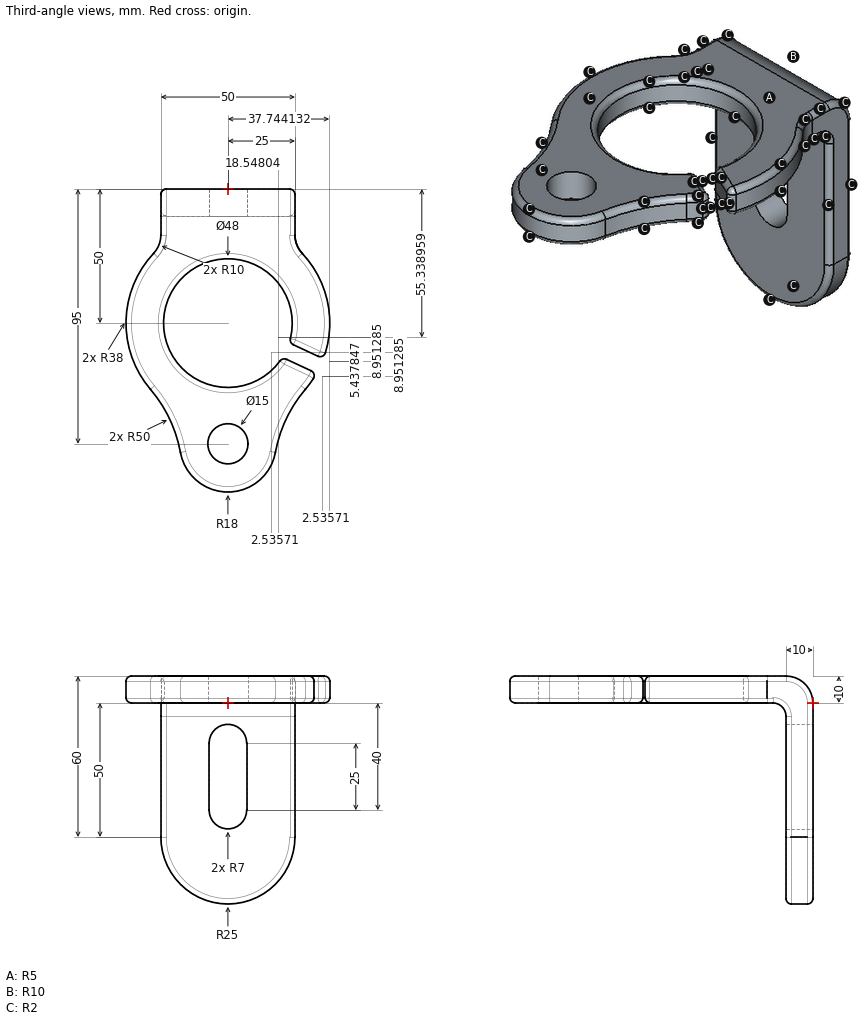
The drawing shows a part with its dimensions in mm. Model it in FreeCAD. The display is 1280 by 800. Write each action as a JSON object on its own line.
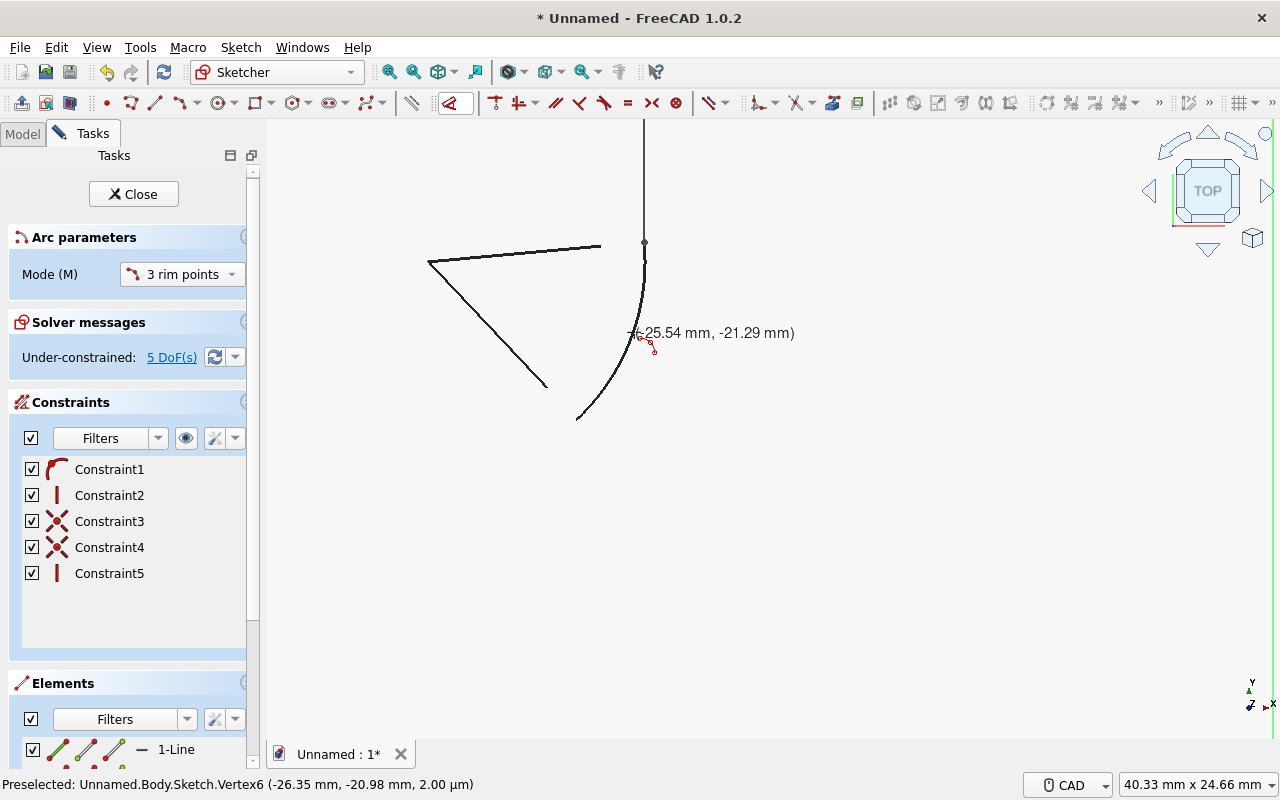
{"action": "left_click", "coordinate": [627, 327]}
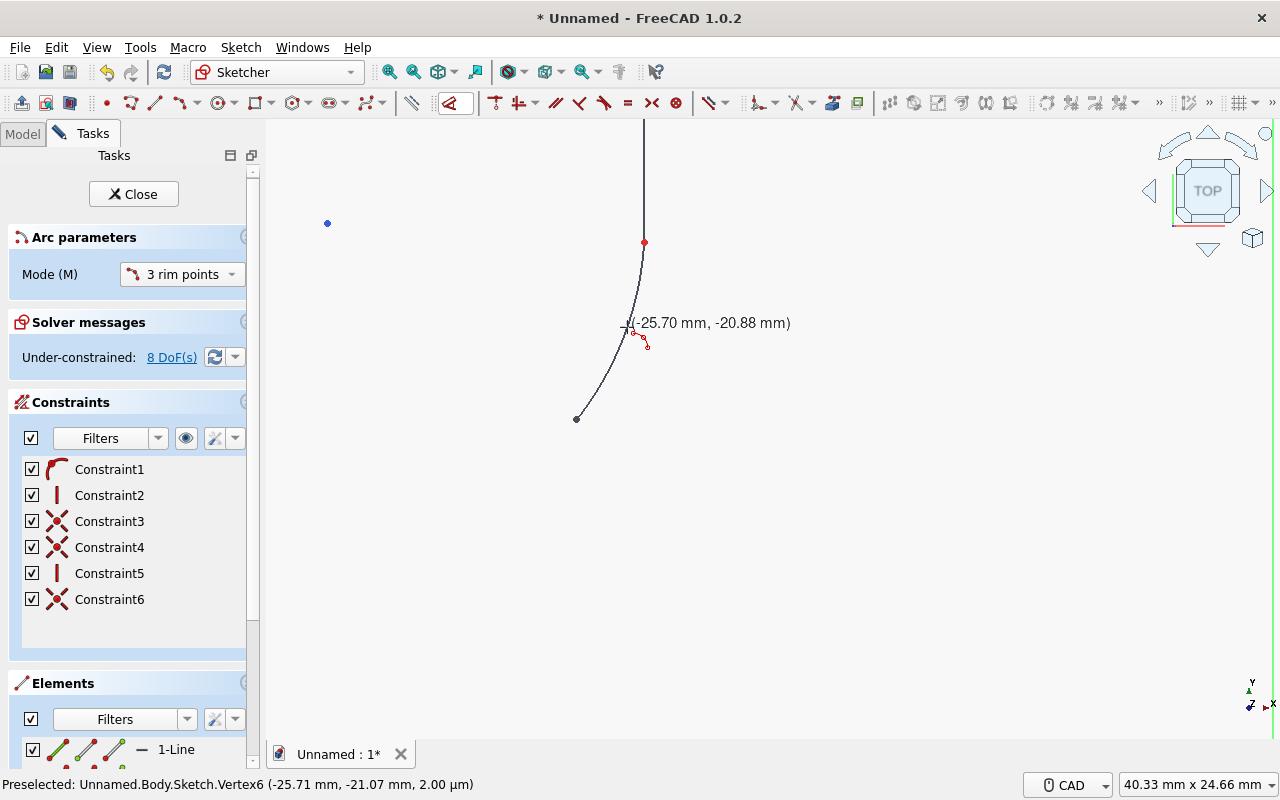
{"action": "scroll", "coordinate": [615, 305], "scroll_direction": "down", "scroll_amount": 10}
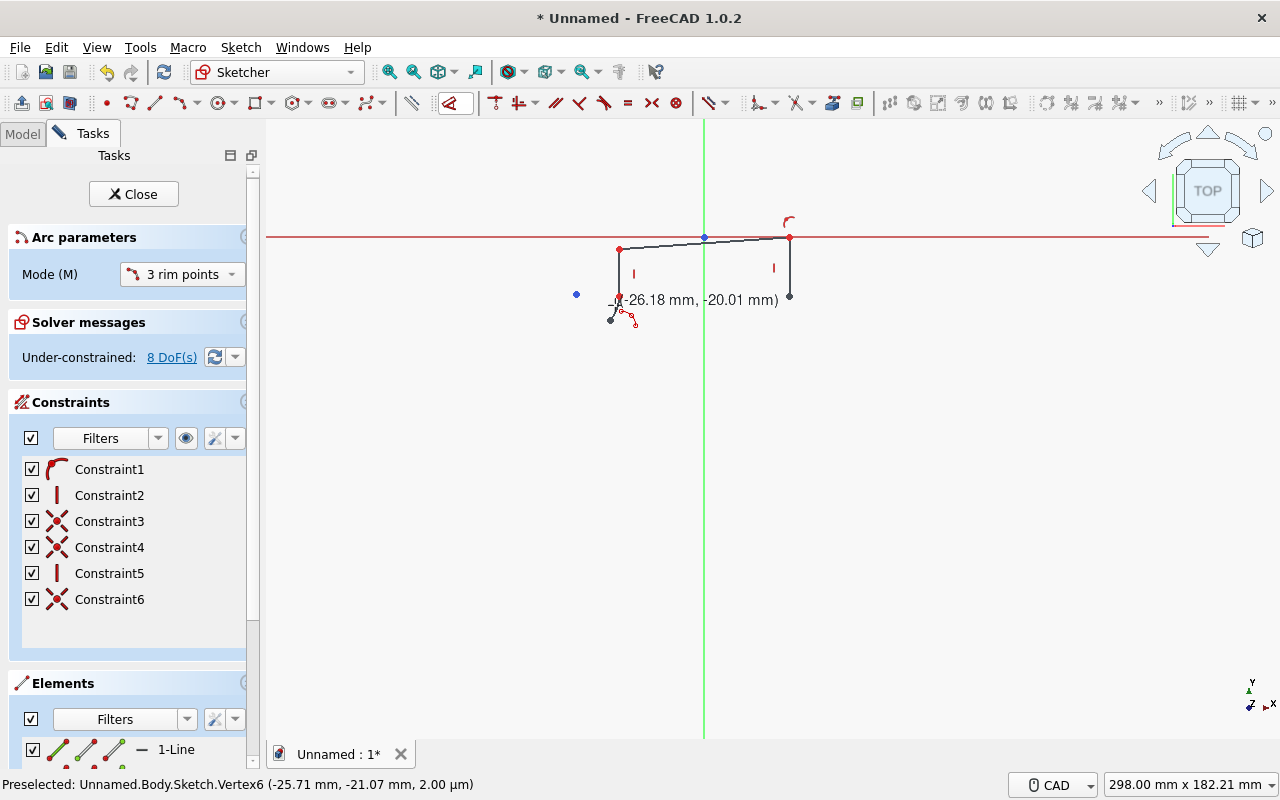
{"action": "left_click", "coordinate": [610, 321]}
{"action": "left_click", "coordinate": [606, 491]}
{"action": "left_click", "coordinate": [575, 404]}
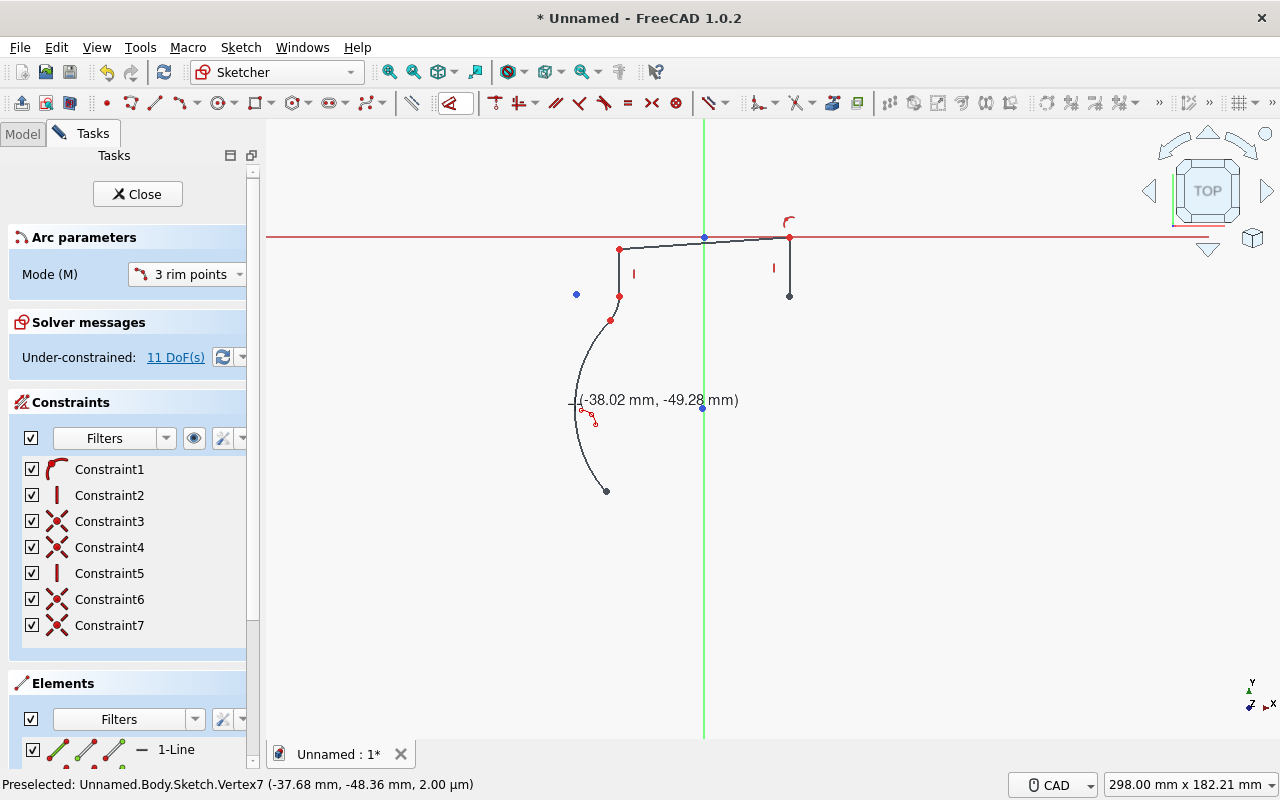
{"action": "left_click", "coordinate": [606, 492]}
{"action": "left_click", "coordinate": [644, 572]}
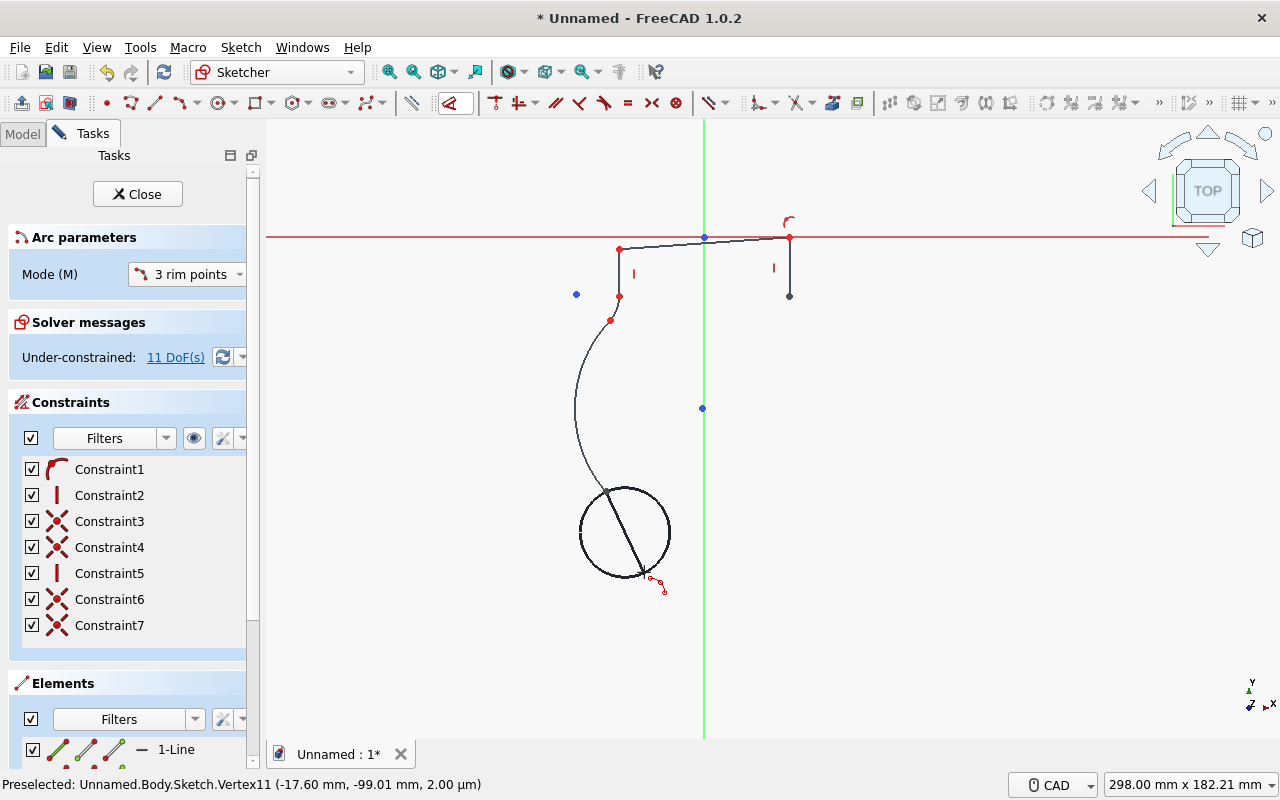
{"action": "scroll", "coordinate": [630, 529], "scroll_direction": "up", "scroll_amount": 5}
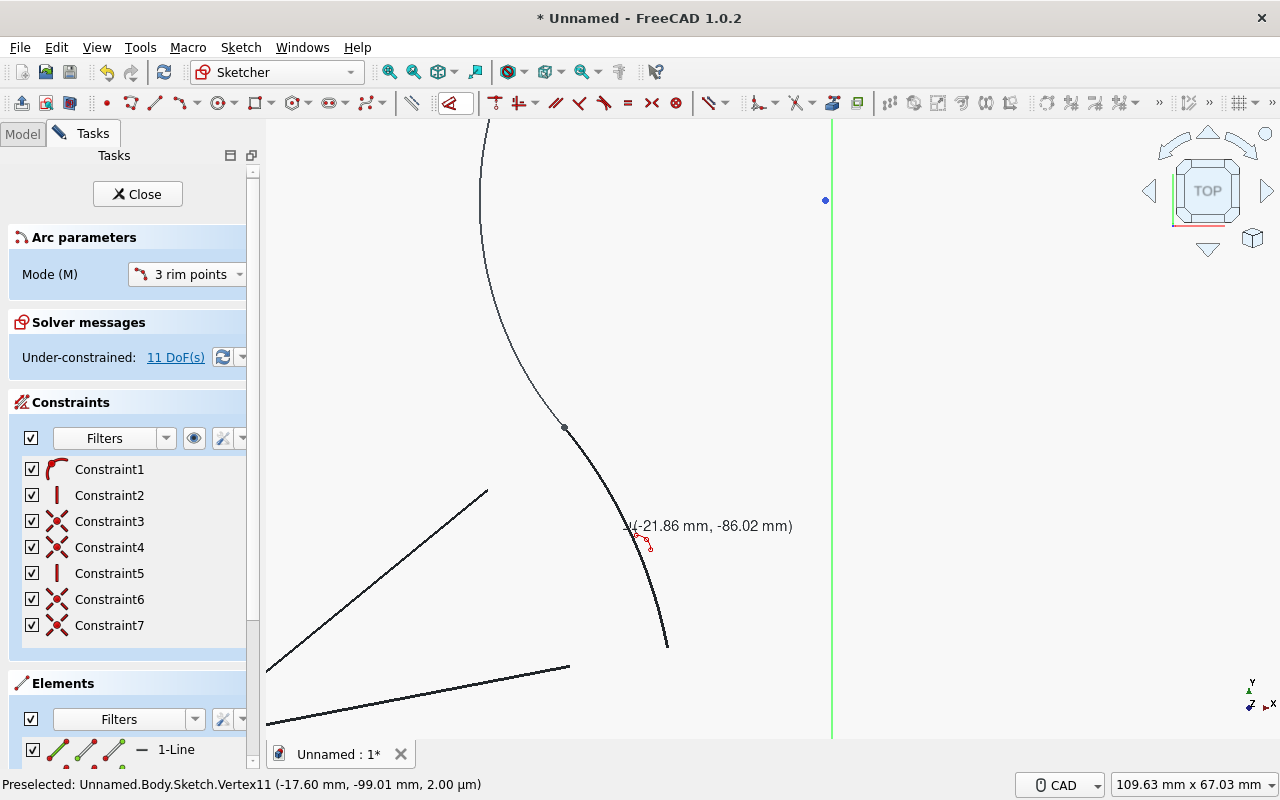
{"action": "left_click", "coordinate": [630, 528]}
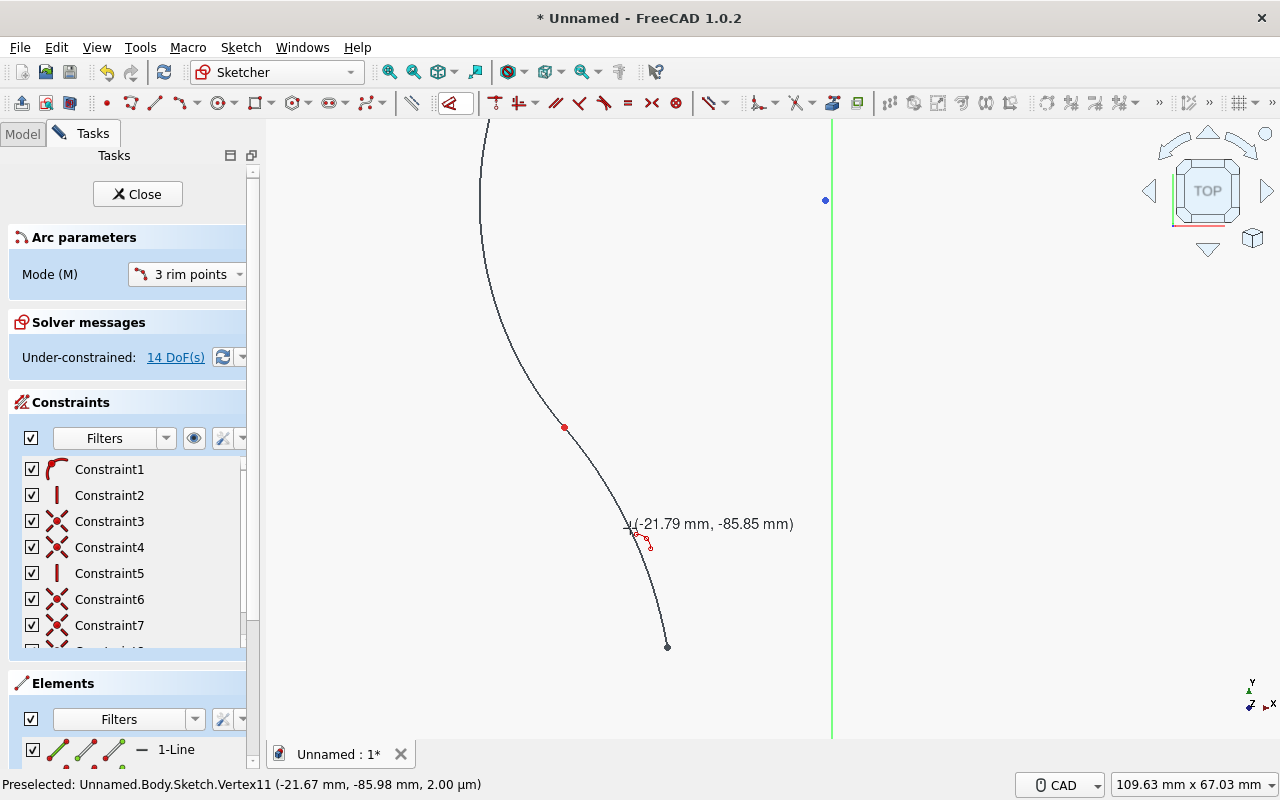
{"action": "left_click", "coordinate": [667, 647]}
{"action": "left_click", "coordinate": [995, 643]}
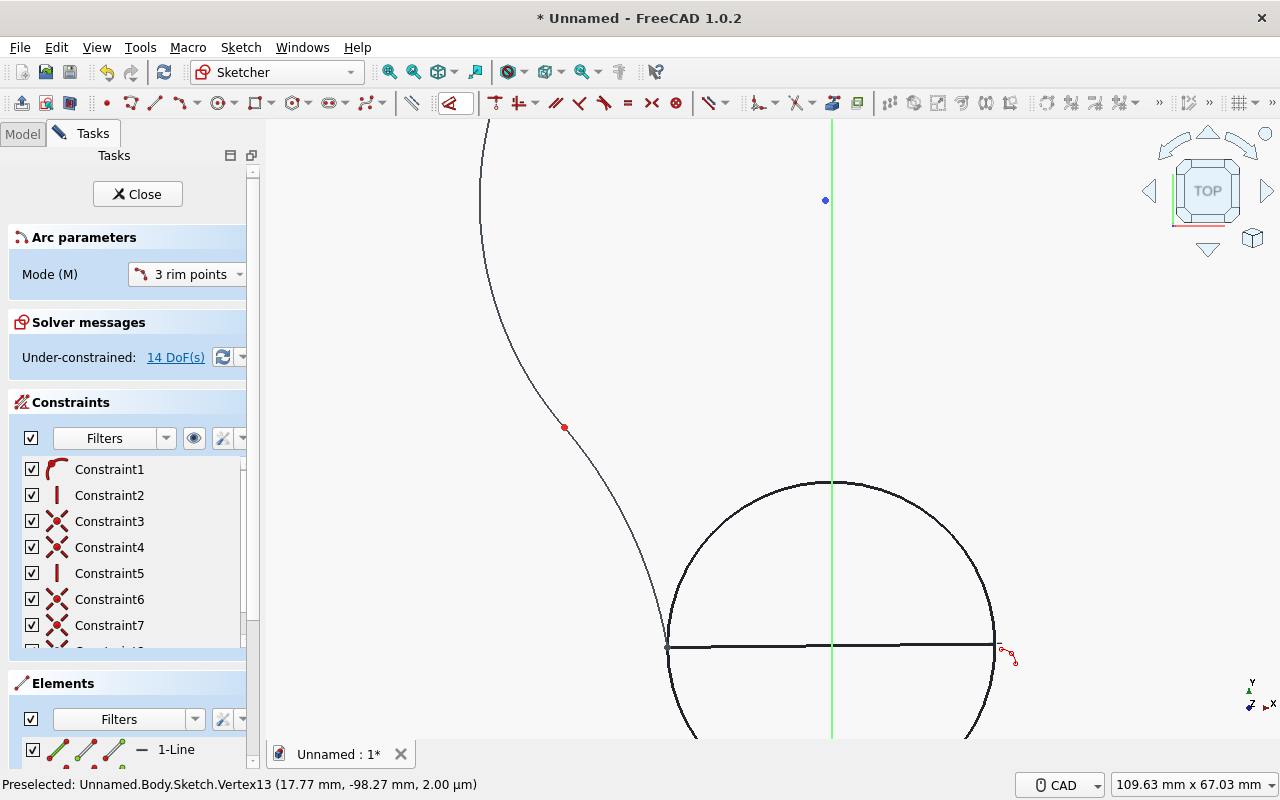
{"action": "scroll", "coordinate": [631, 529], "scroll_direction": "down", "scroll_amount": 5}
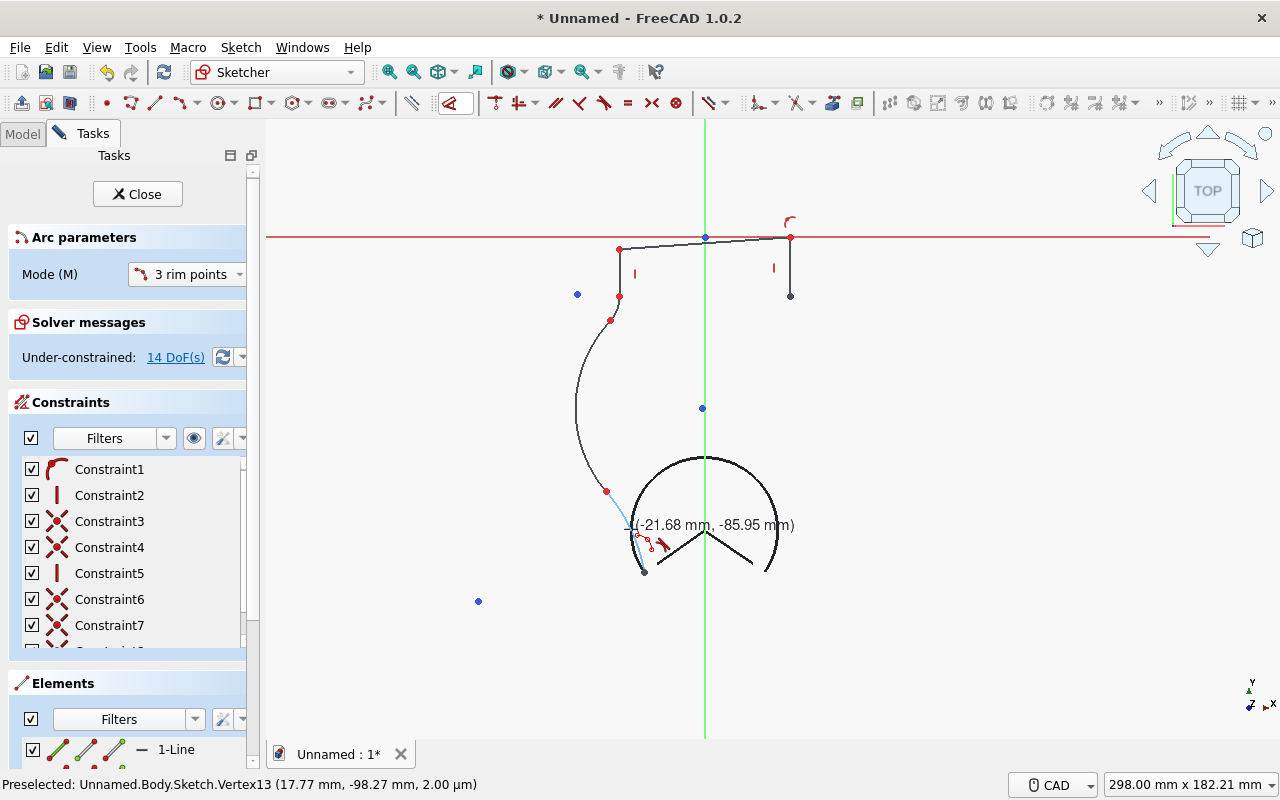
{"action": "left_click", "coordinate": [673, 613]}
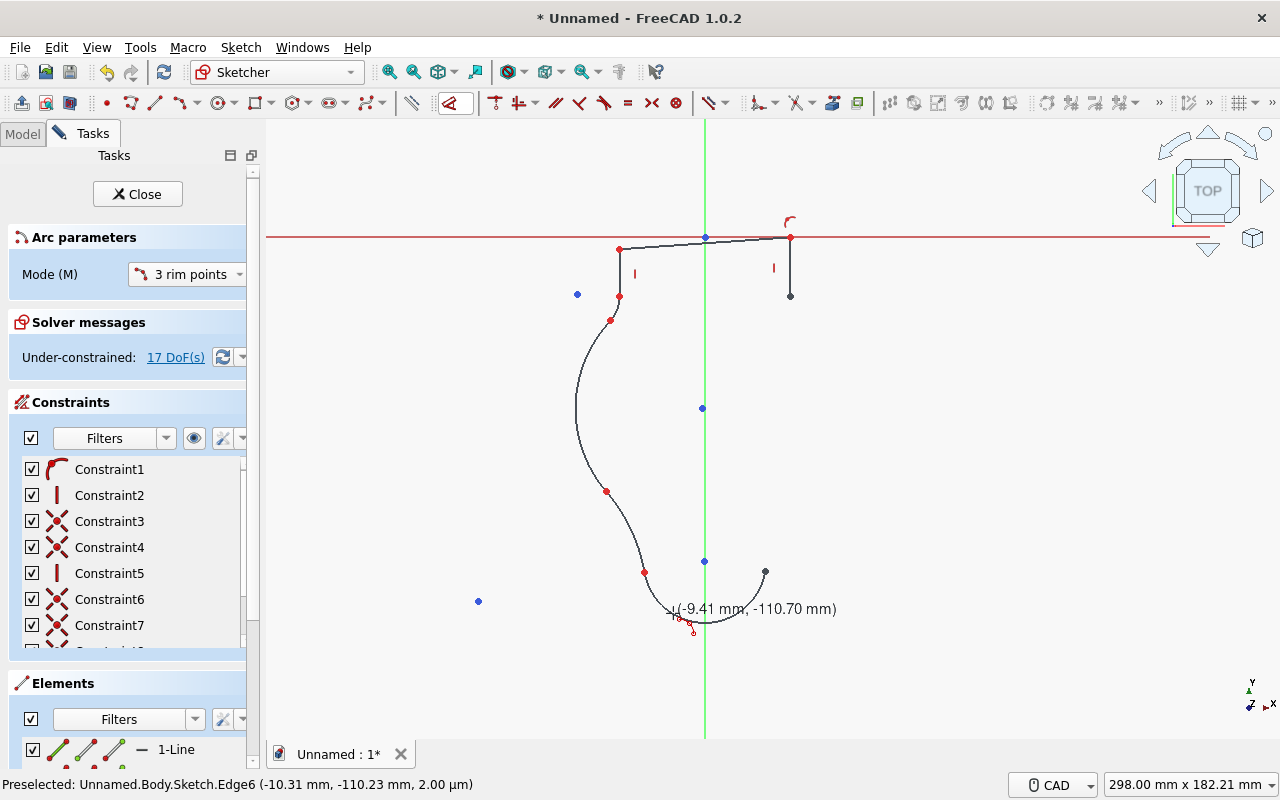
{"action": "left_click", "coordinate": [765, 572]}
{"action": "left_click", "coordinate": [803, 491]}